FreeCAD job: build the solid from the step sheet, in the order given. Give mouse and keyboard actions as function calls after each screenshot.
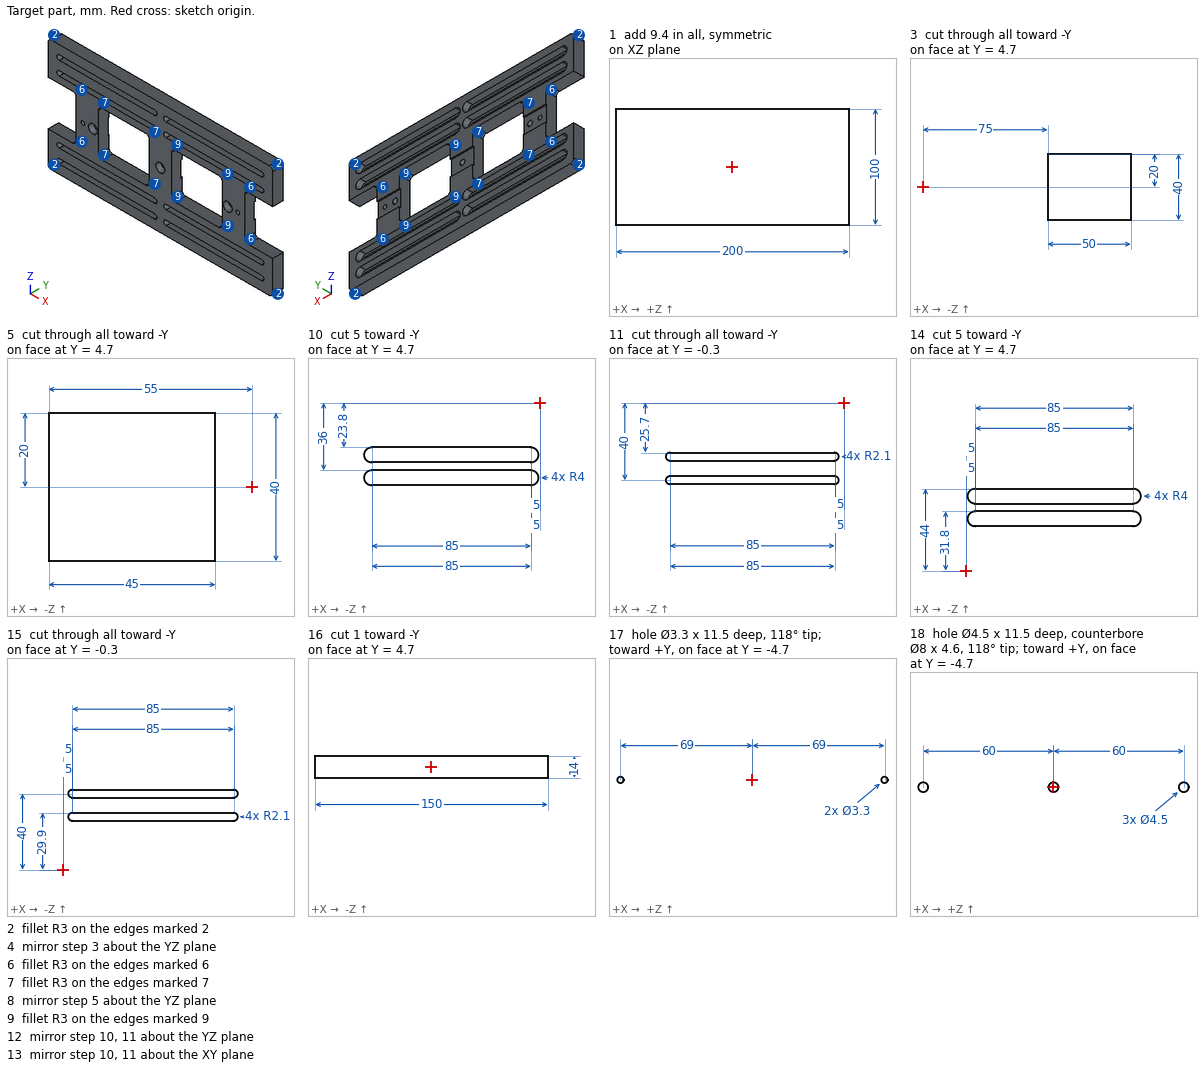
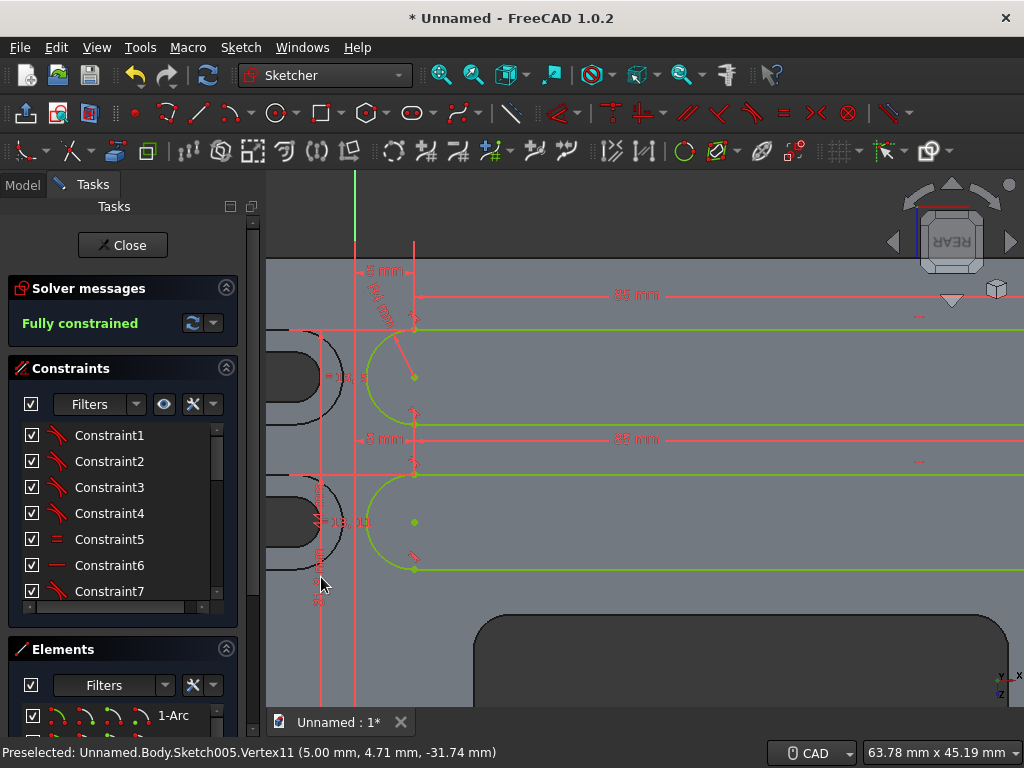
click(123, 245)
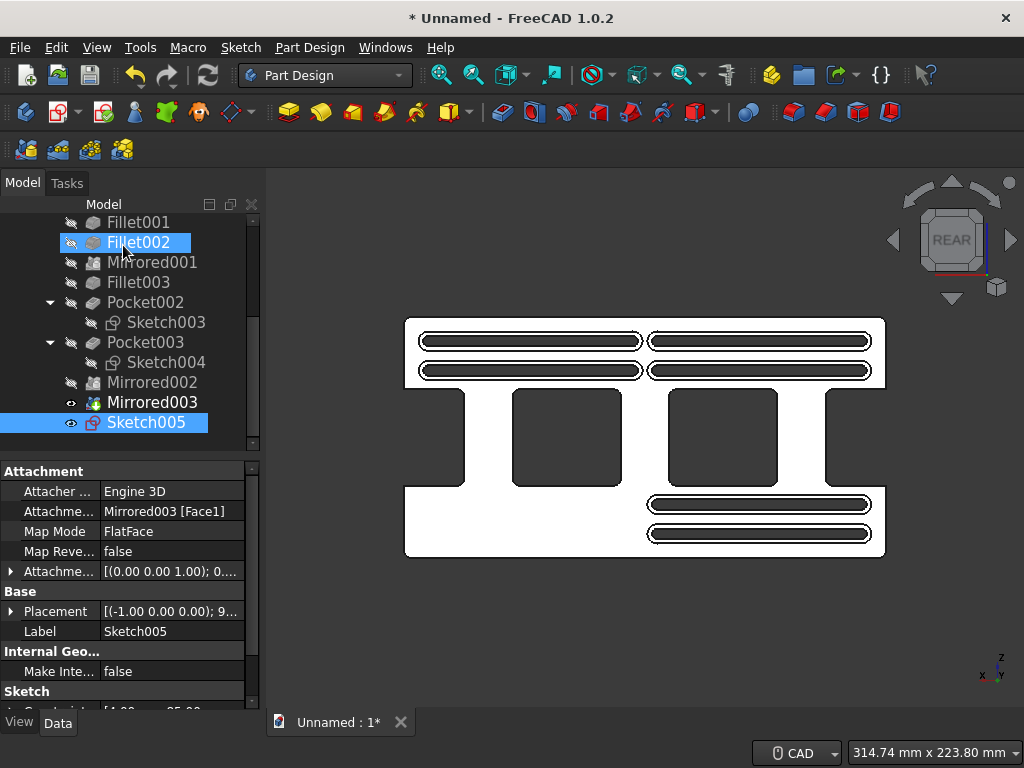
click(504, 112)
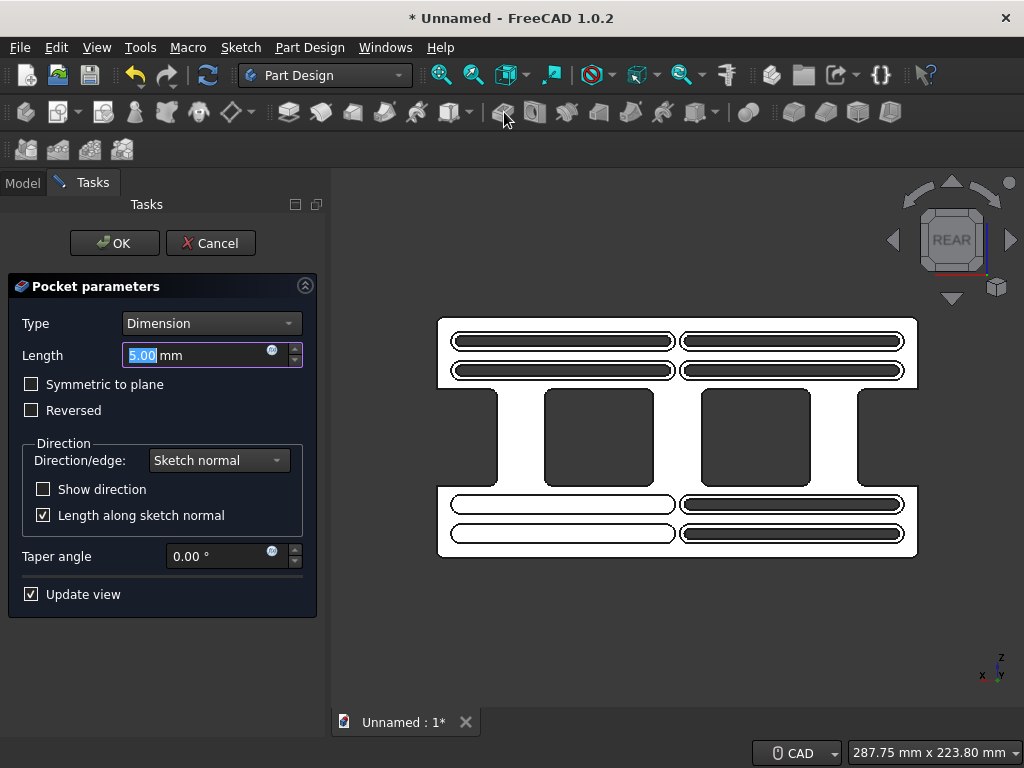
text(5)
key(Tab)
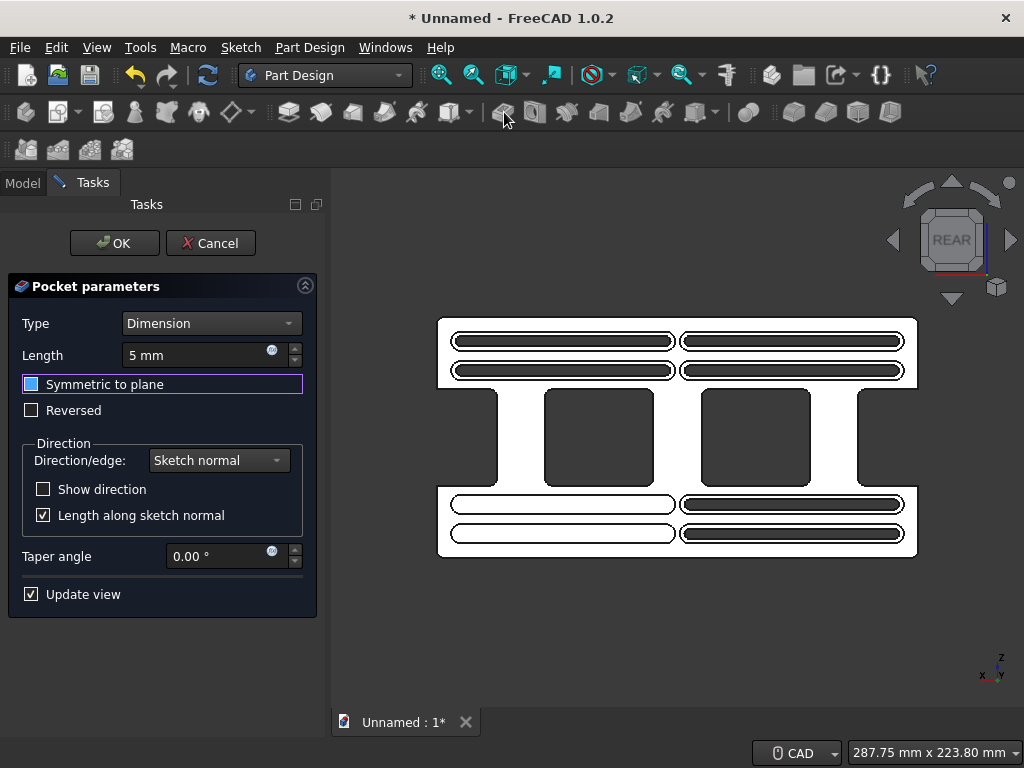
click(115, 243)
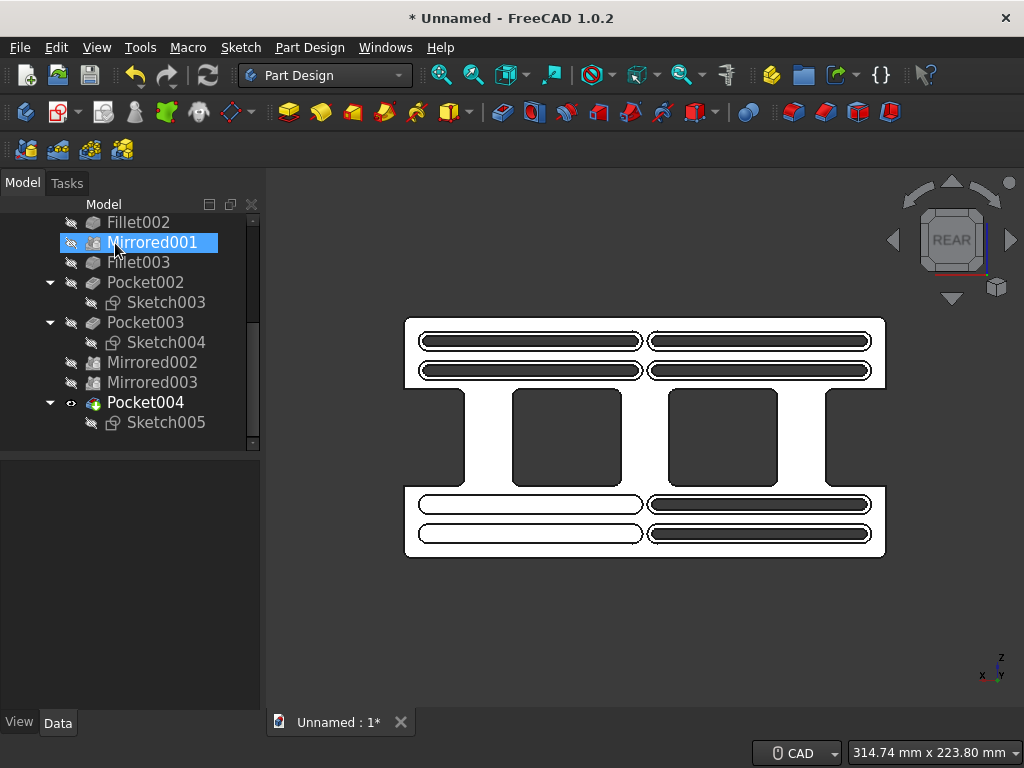
click(435, 503)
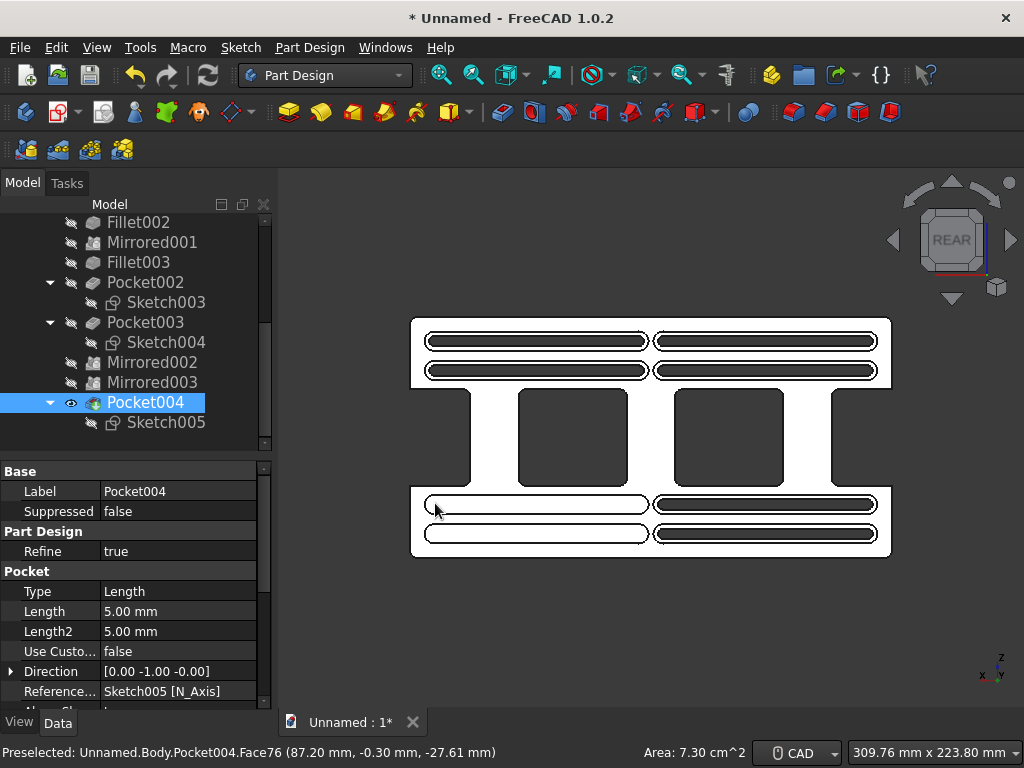
click(58, 112)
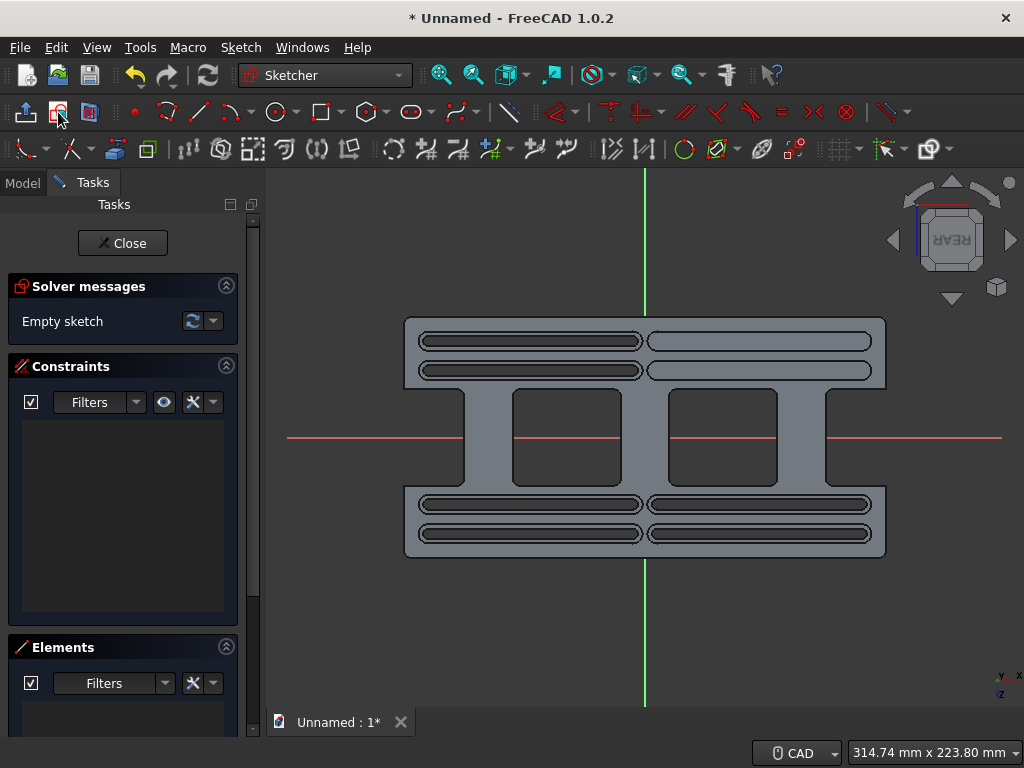
scroll(576, 438, down, 5)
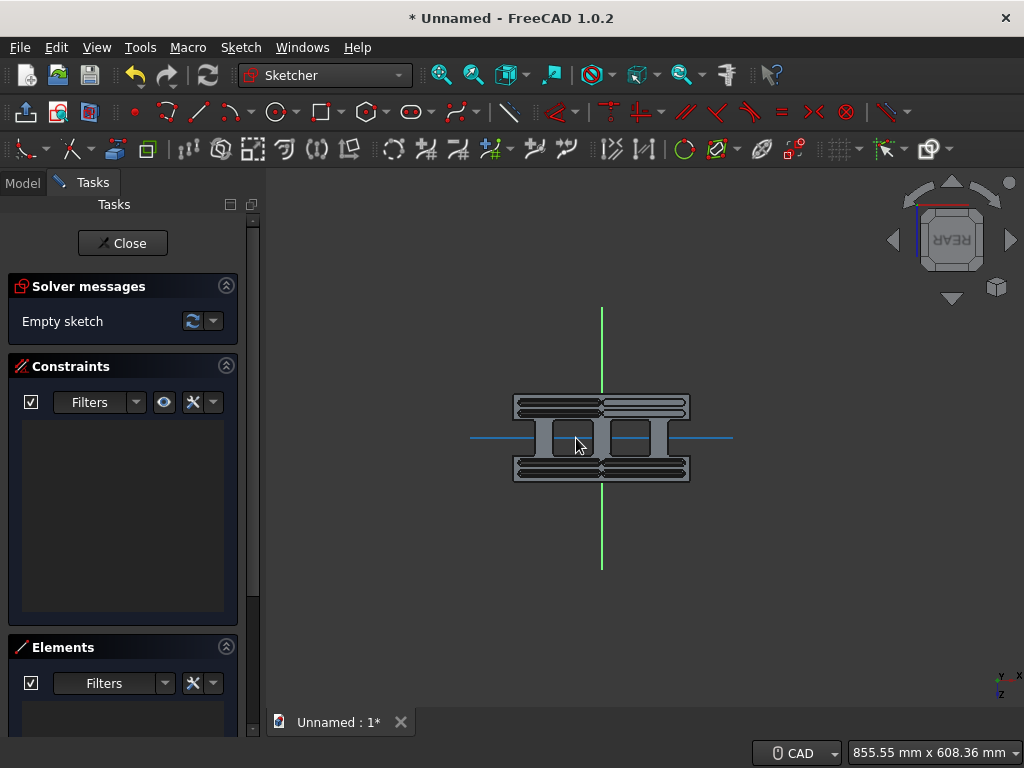
scroll(659, 415, up, 8)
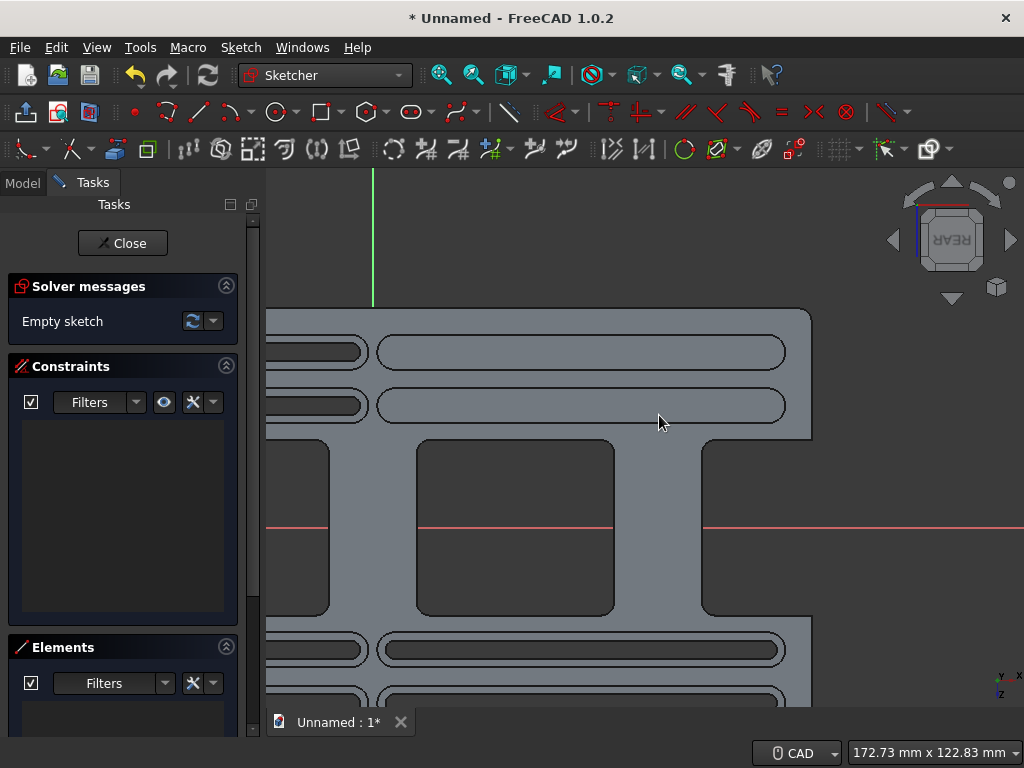
key(g)
key(s)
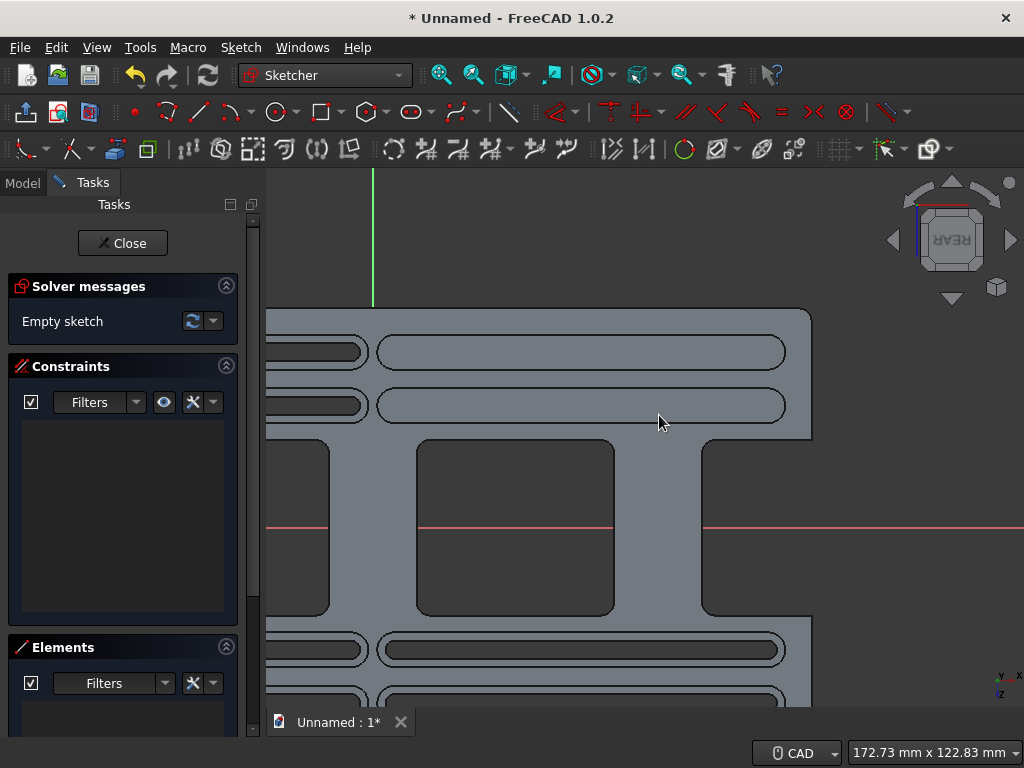
scroll(395, 406, up, 5)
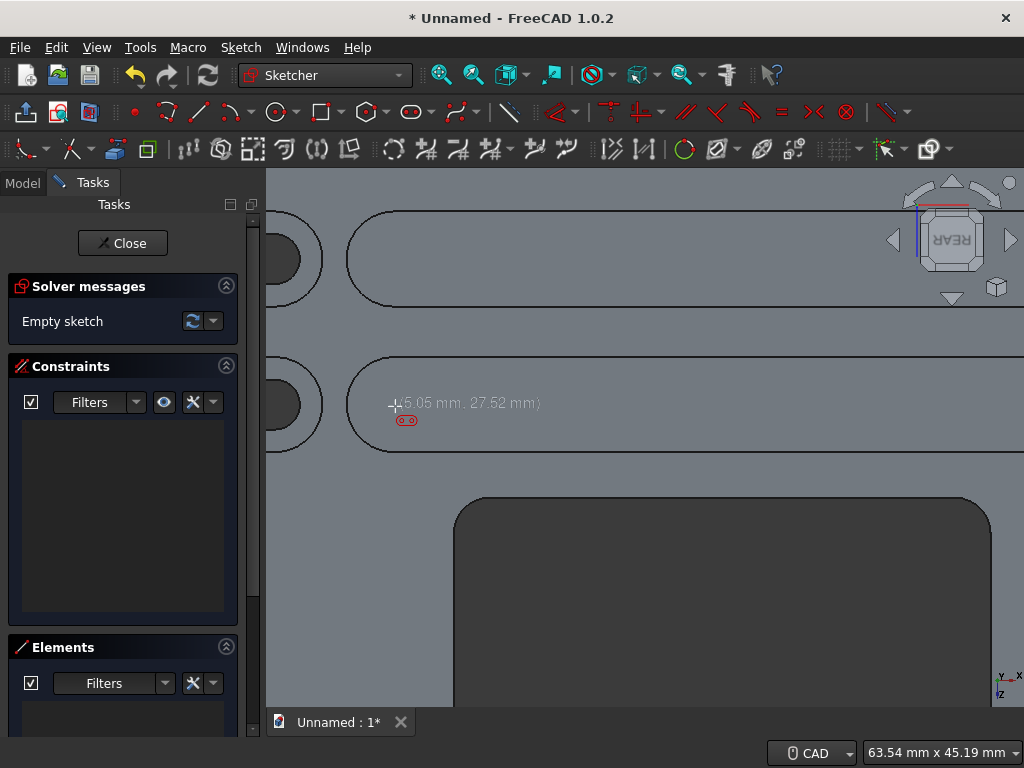
click(394, 405)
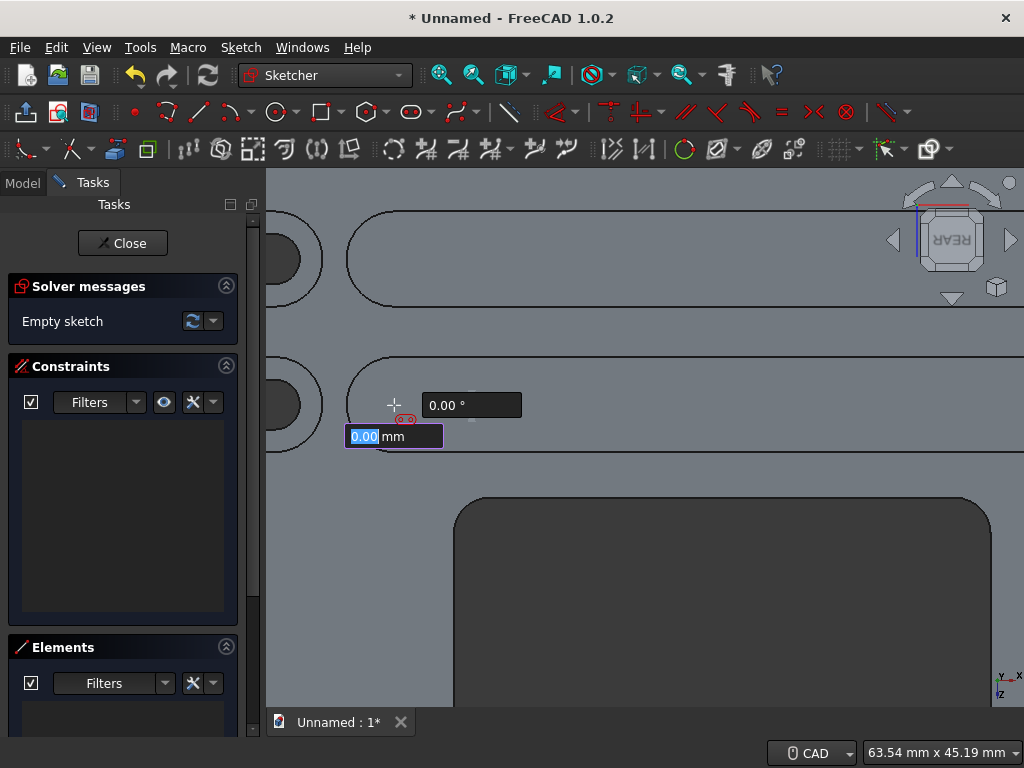
scroll(398, 410, down, 5)